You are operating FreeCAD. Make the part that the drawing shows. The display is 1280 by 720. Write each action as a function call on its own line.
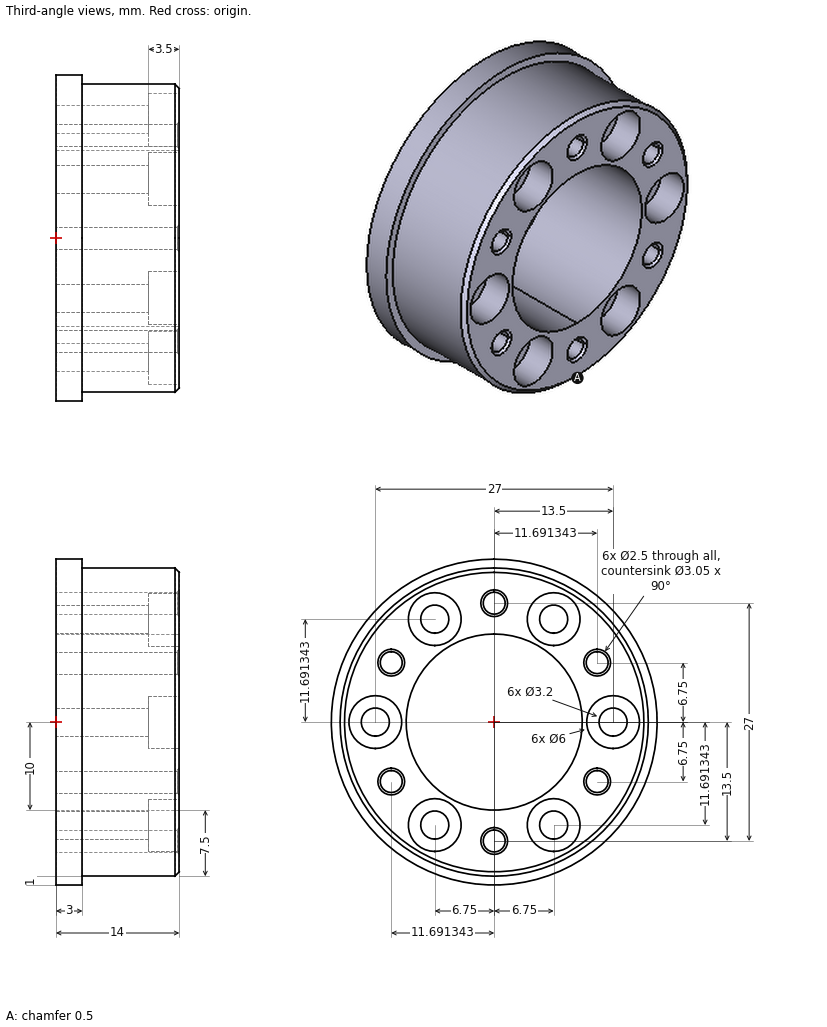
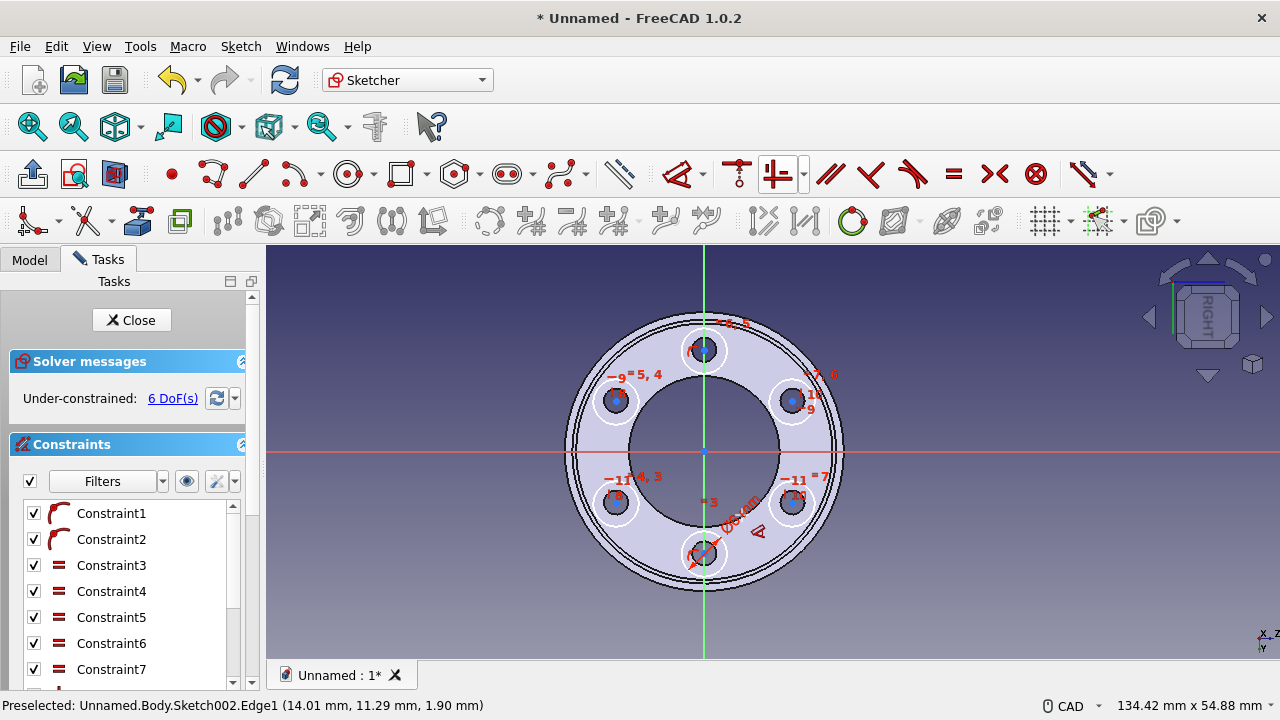
click(704, 554)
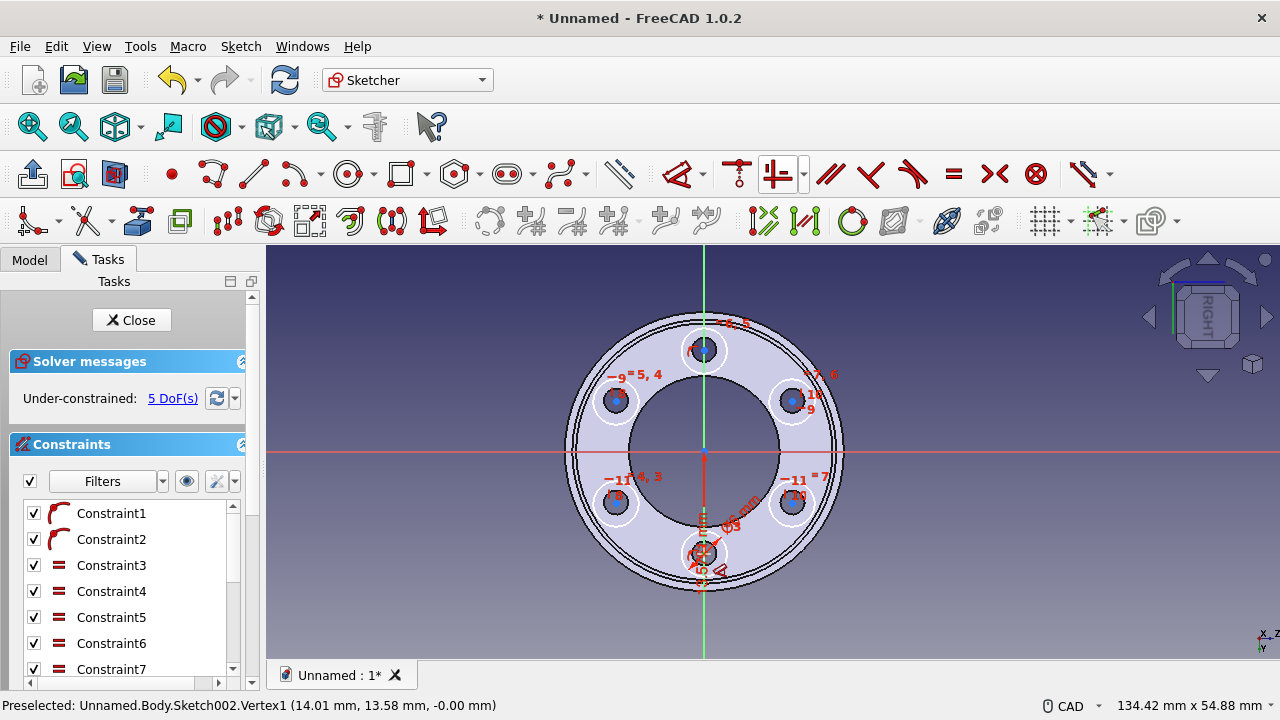
click(704, 351)
click(738, 406)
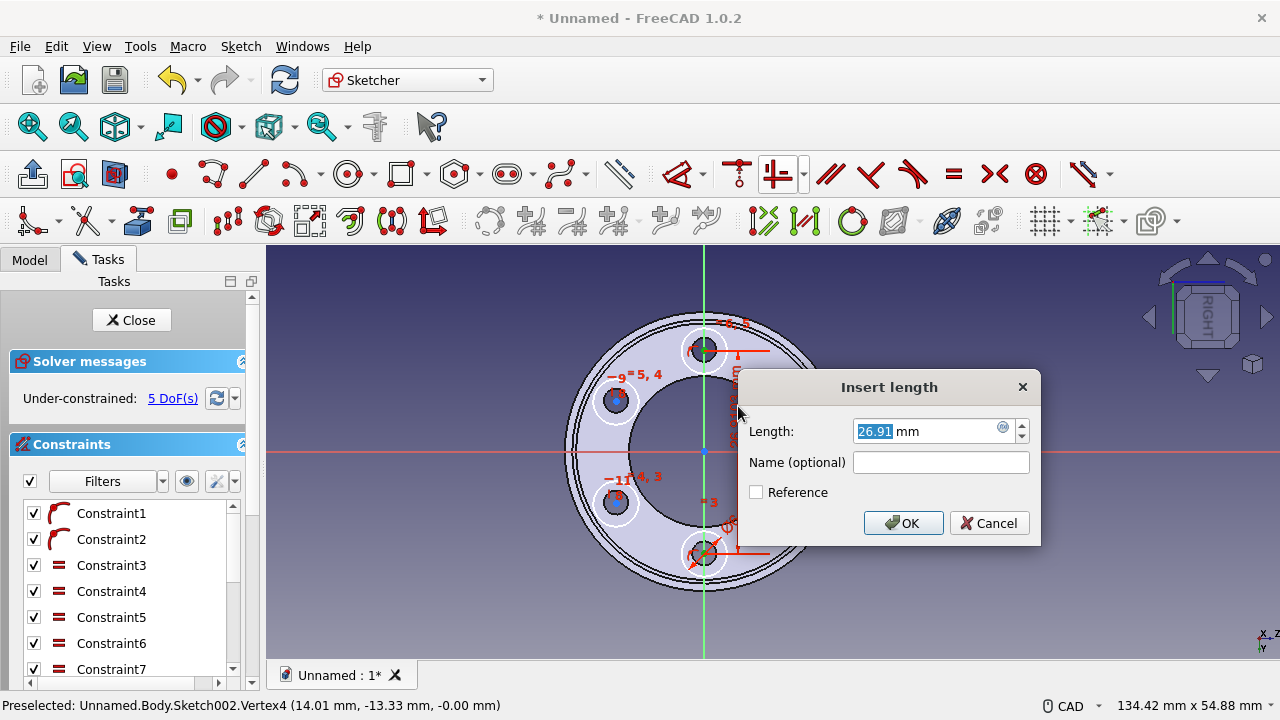
text(27)
key(Return)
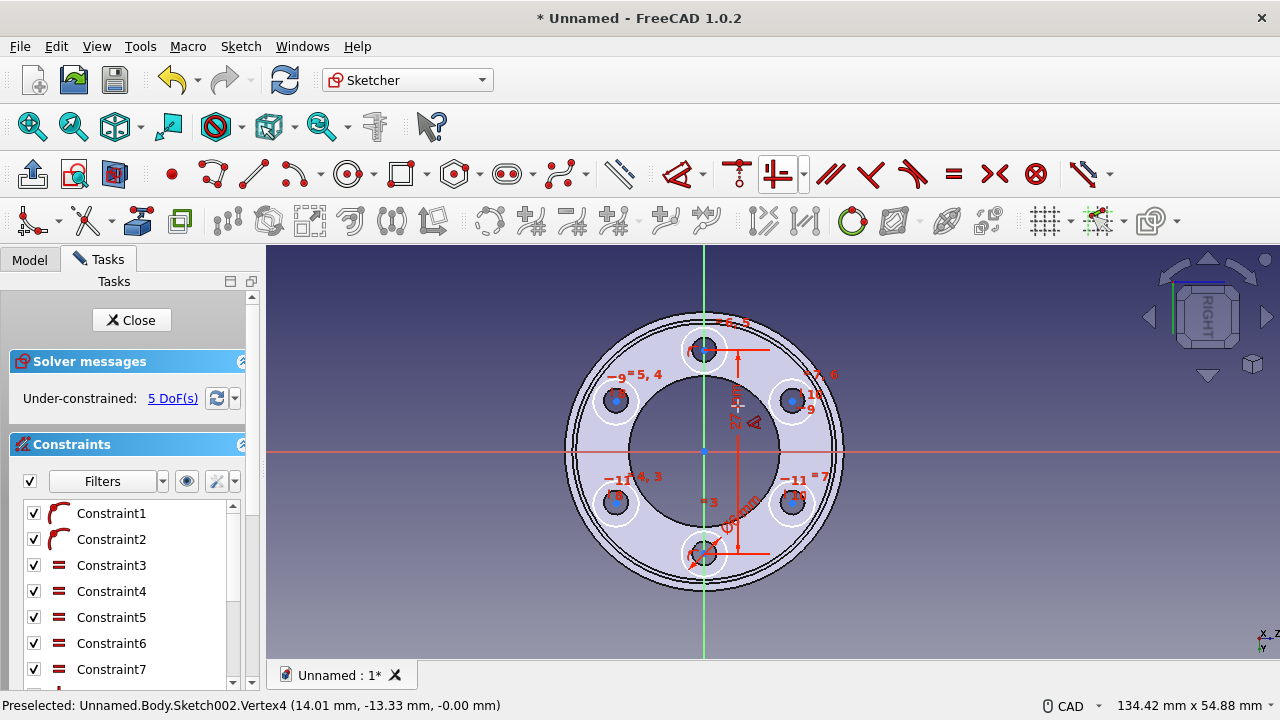
click(704, 554)
click(738, 479)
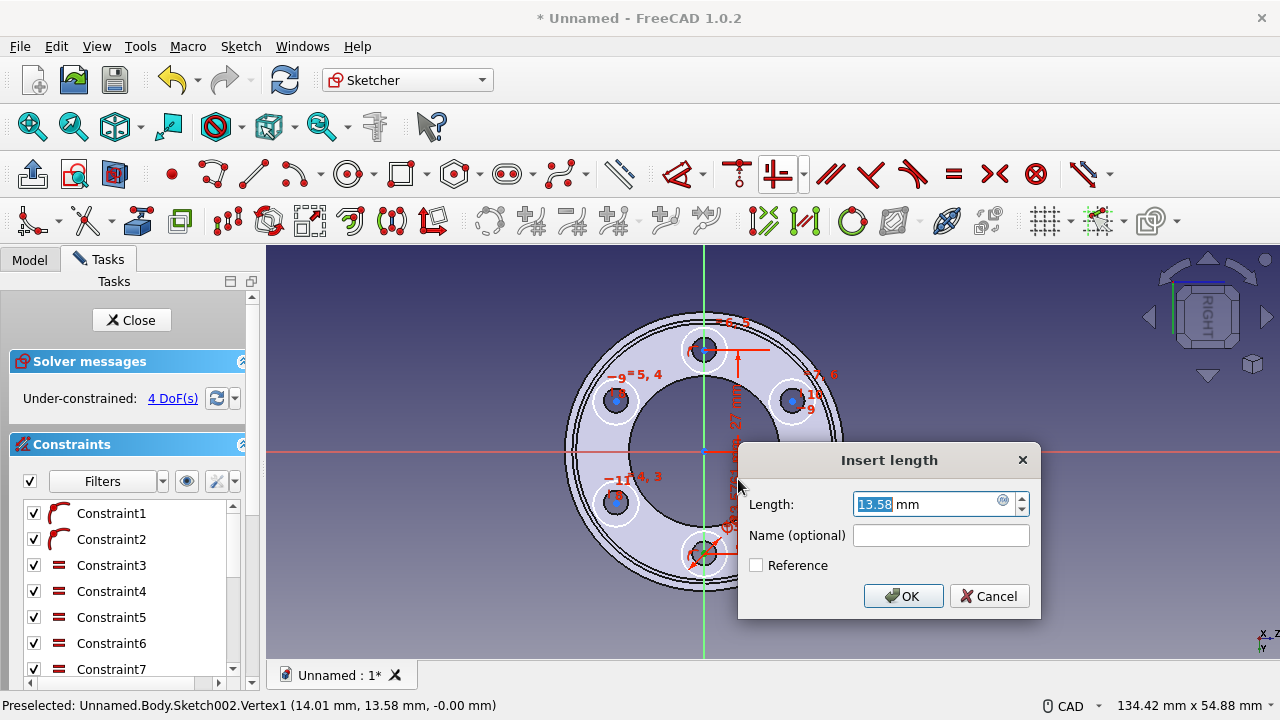
text(13.5)
key(Return)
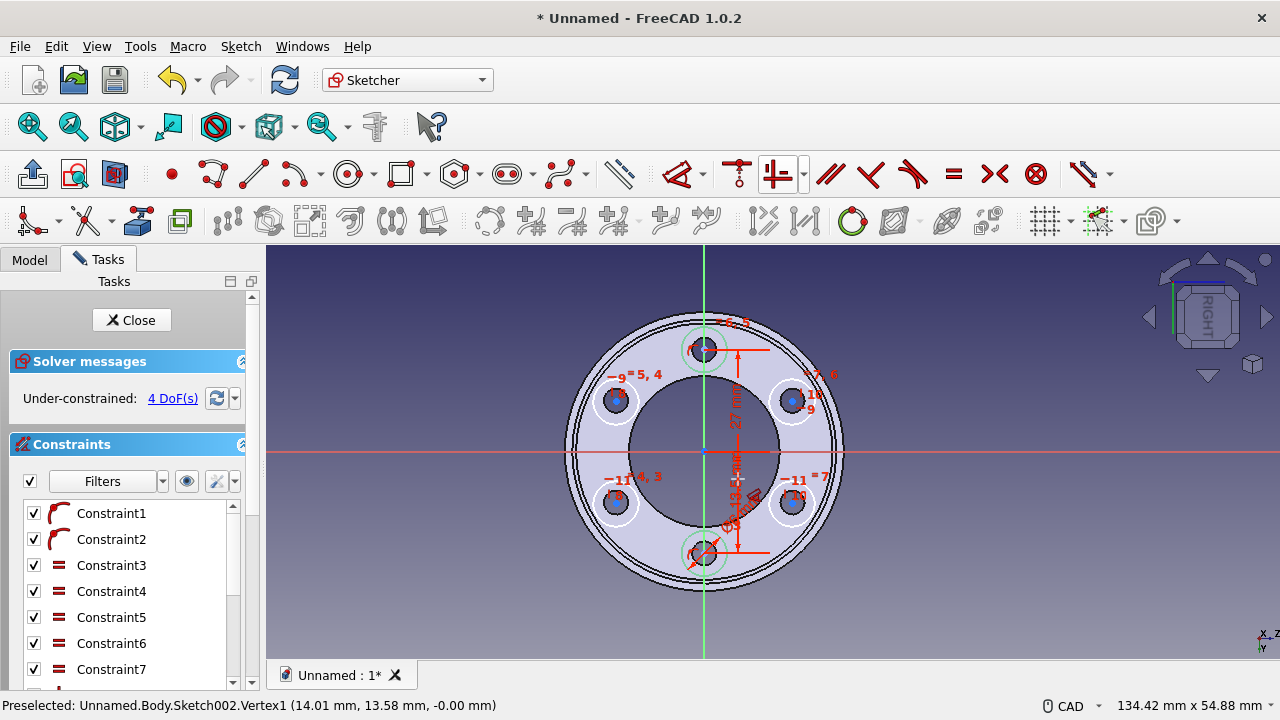
click(616, 504)
click(582, 478)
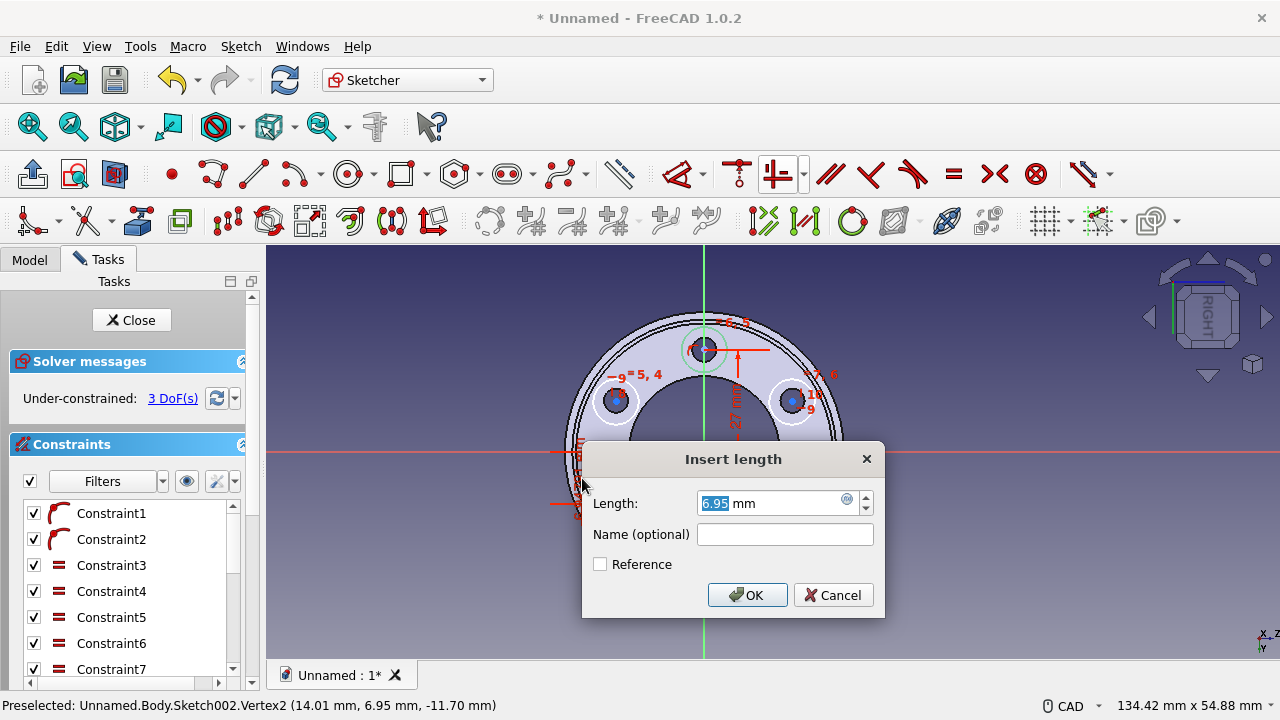
text(6.75)
key(Return)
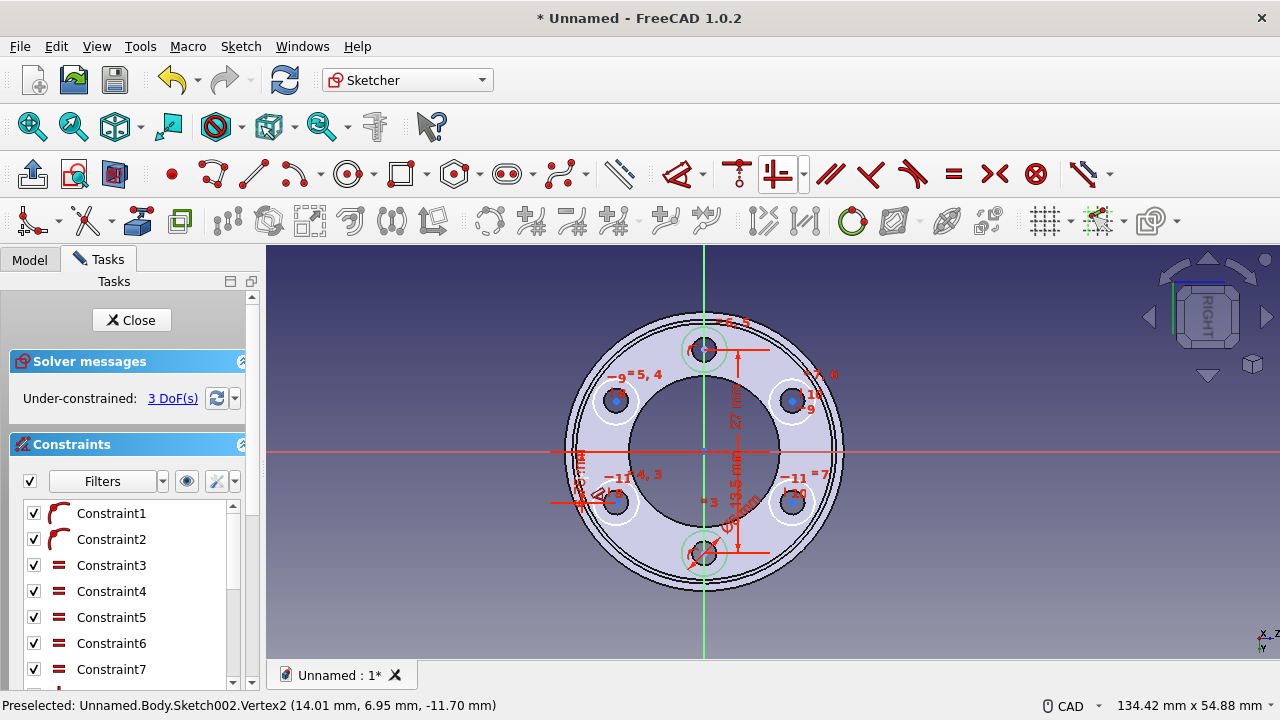
click(616, 402)
click(582, 427)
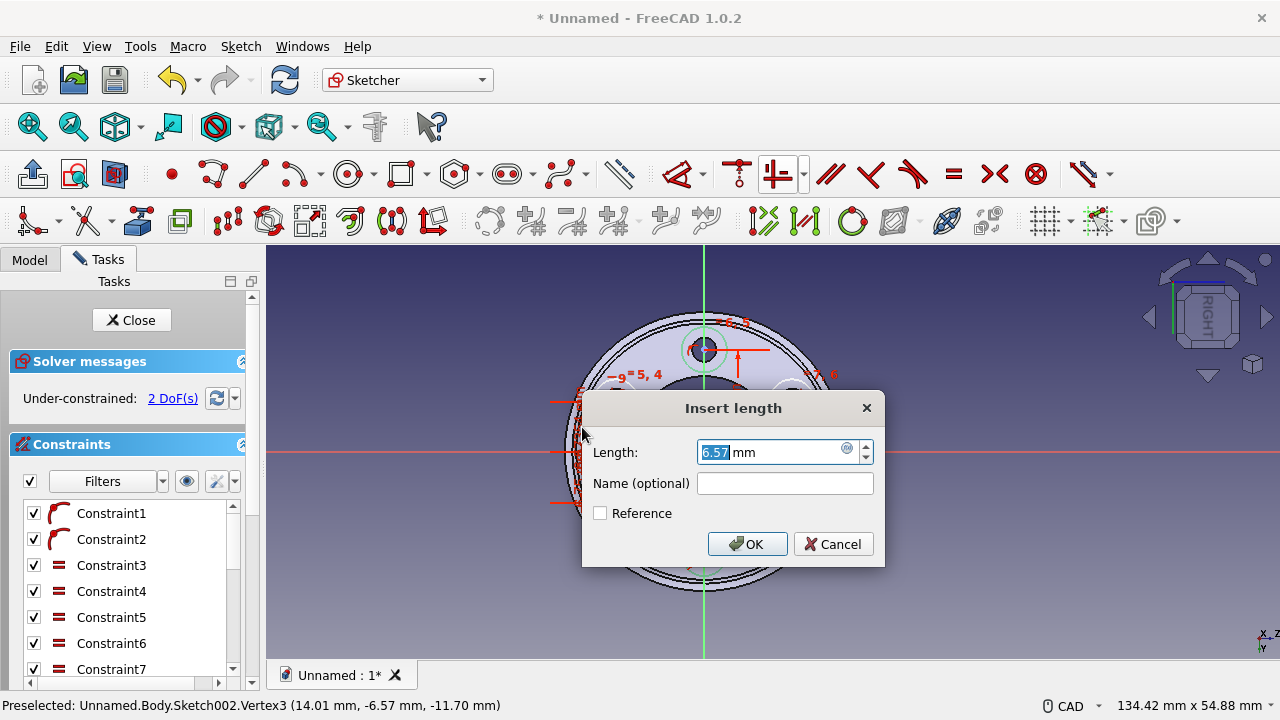
text(6.75)
key(Return)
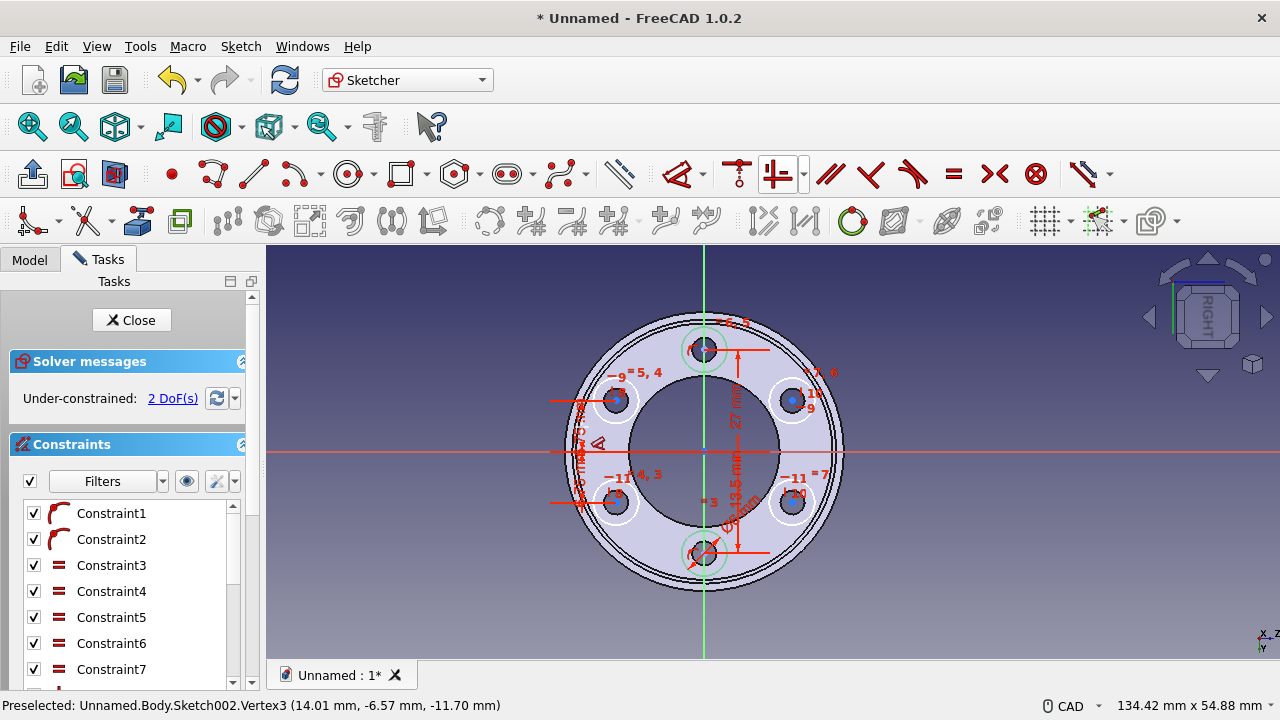
click(616, 503)
click(660, 537)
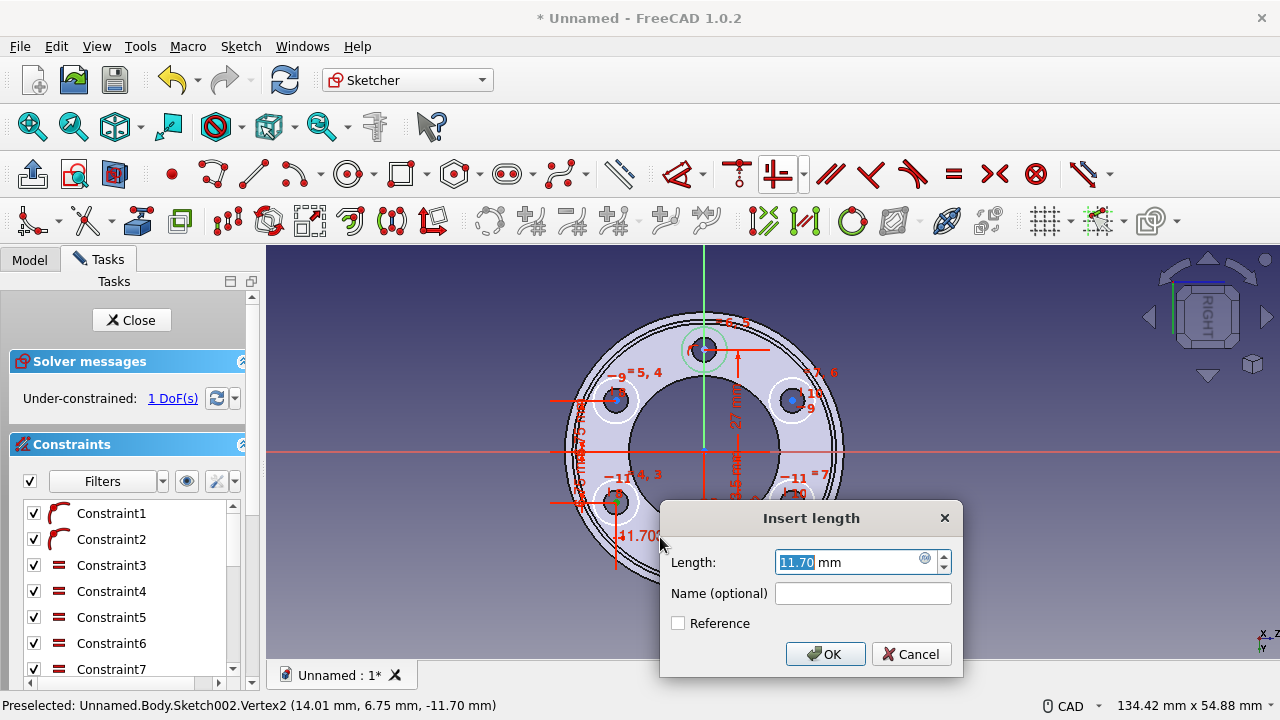
text(11.691343)
key(Return)